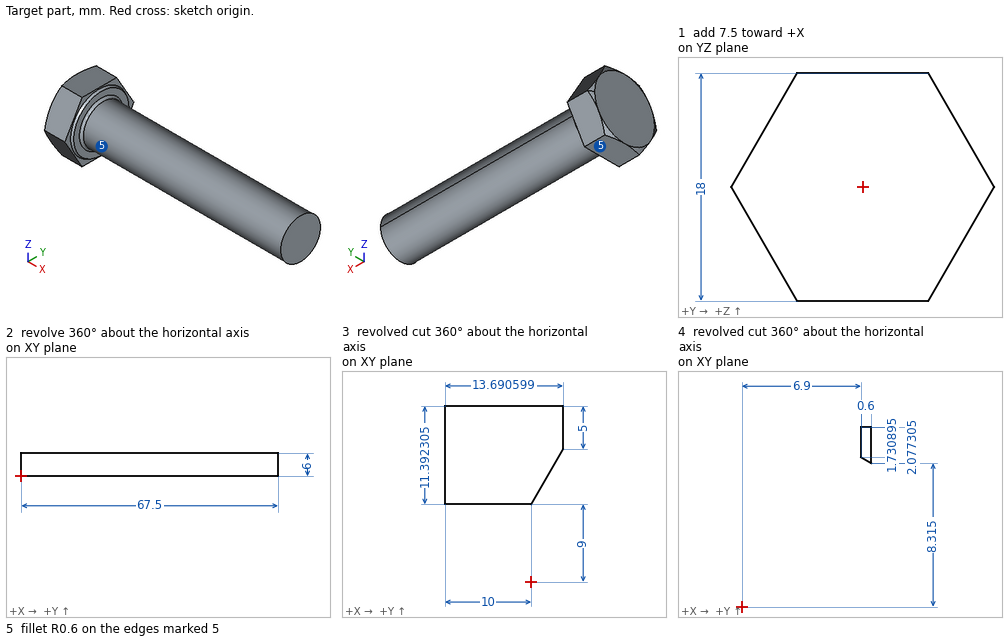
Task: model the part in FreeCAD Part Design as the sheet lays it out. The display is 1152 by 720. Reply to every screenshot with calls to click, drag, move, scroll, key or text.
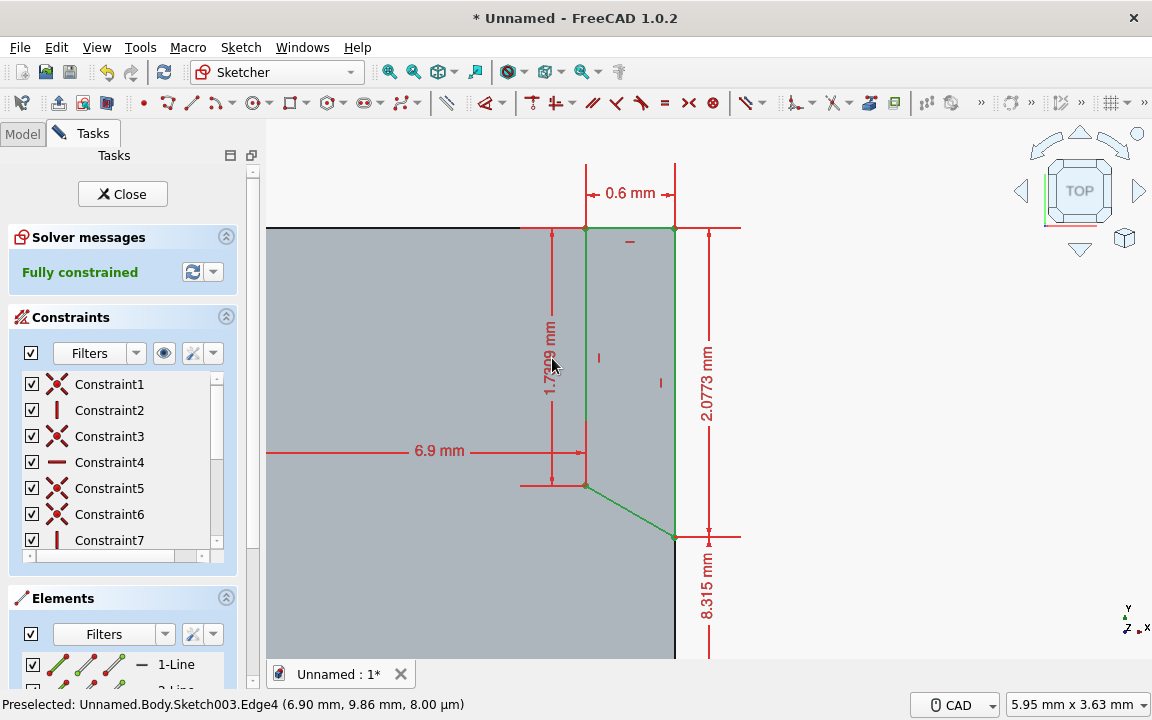
click(123, 194)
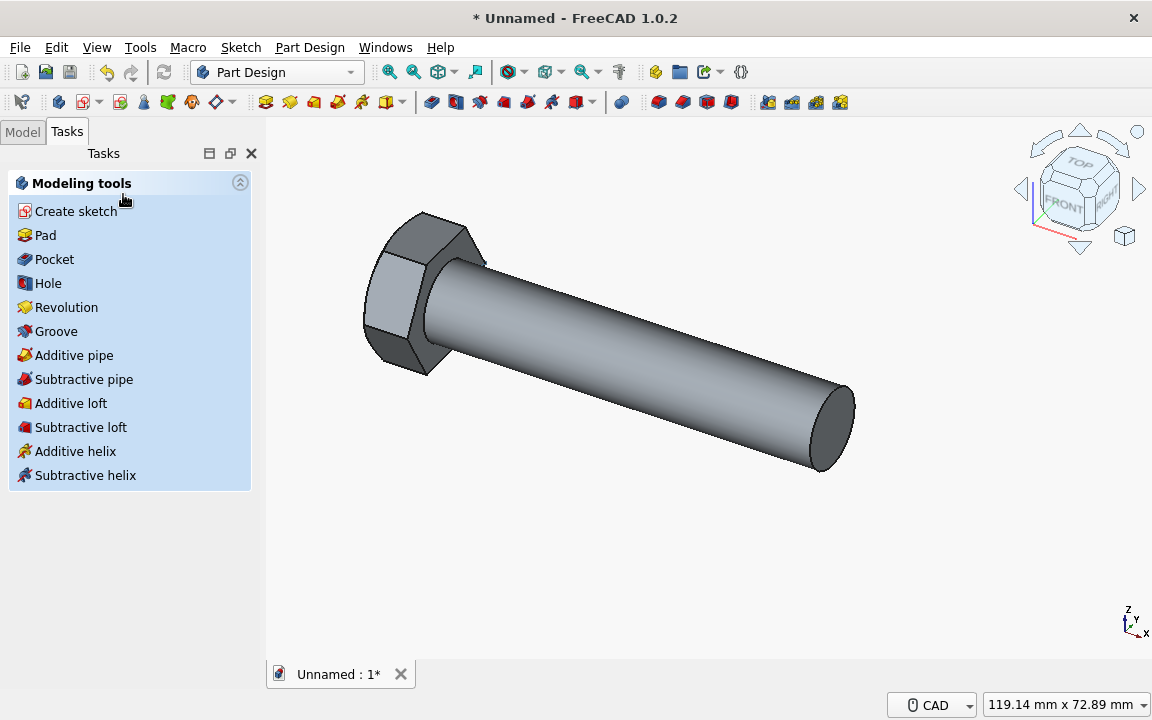
click(480, 102)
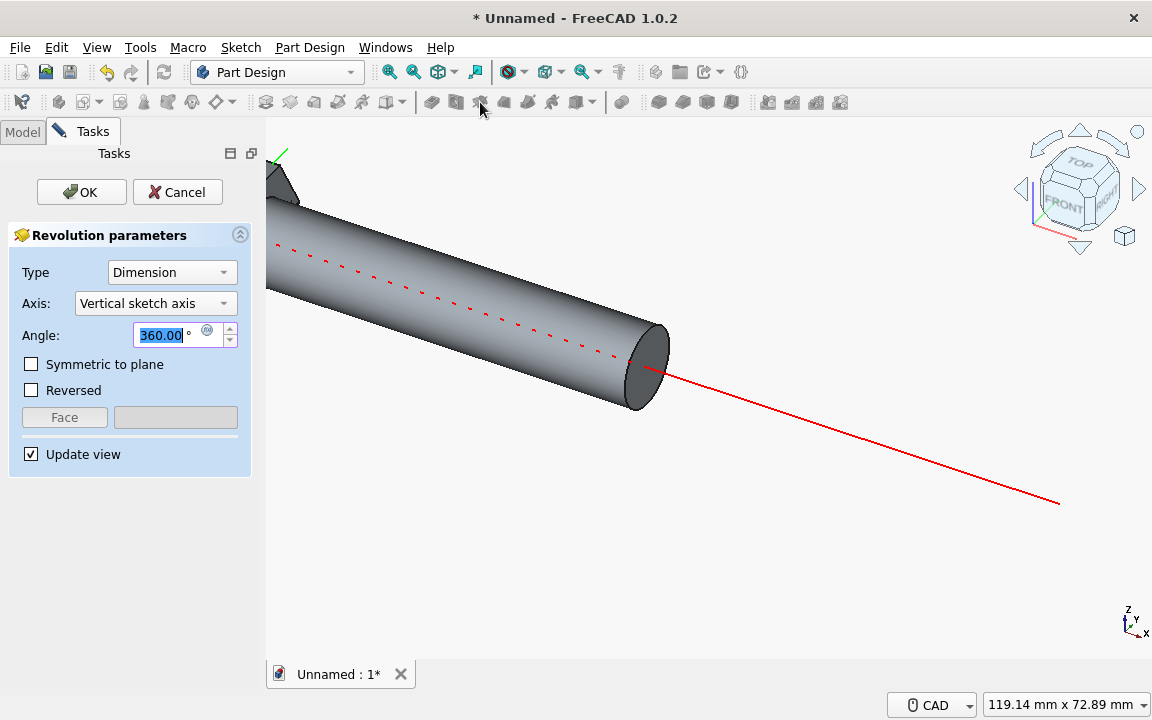
click(156, 304)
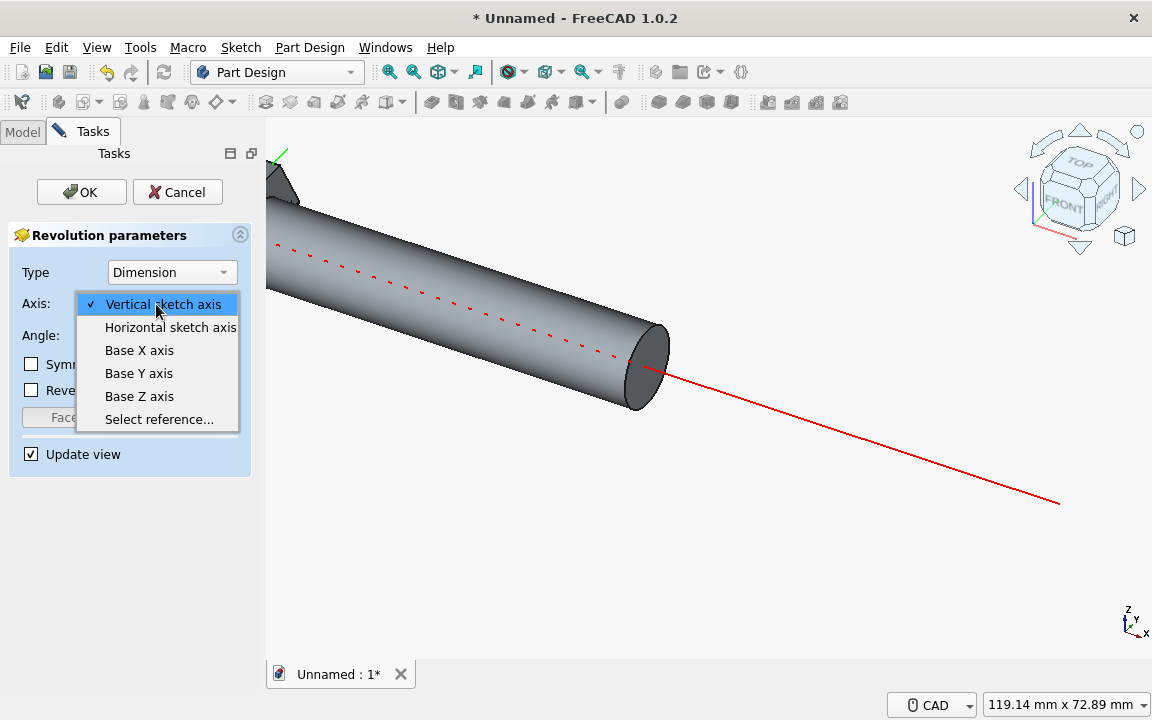
click(156, 328)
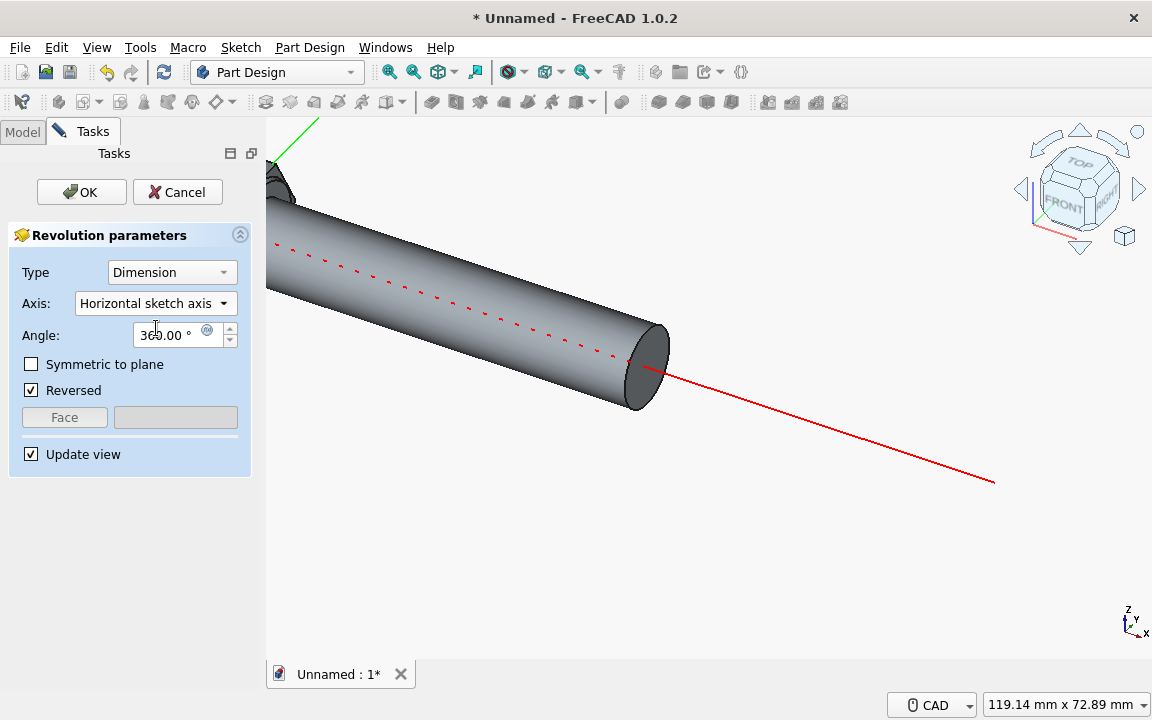
click(82, 192)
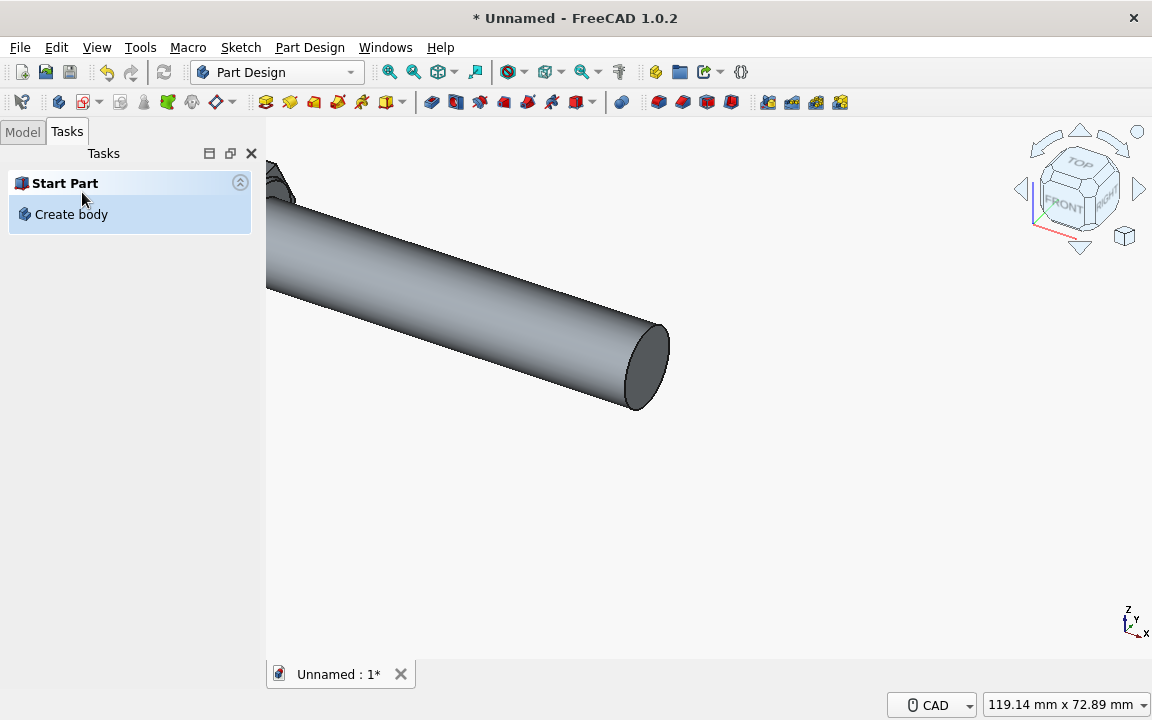
click(390, 72)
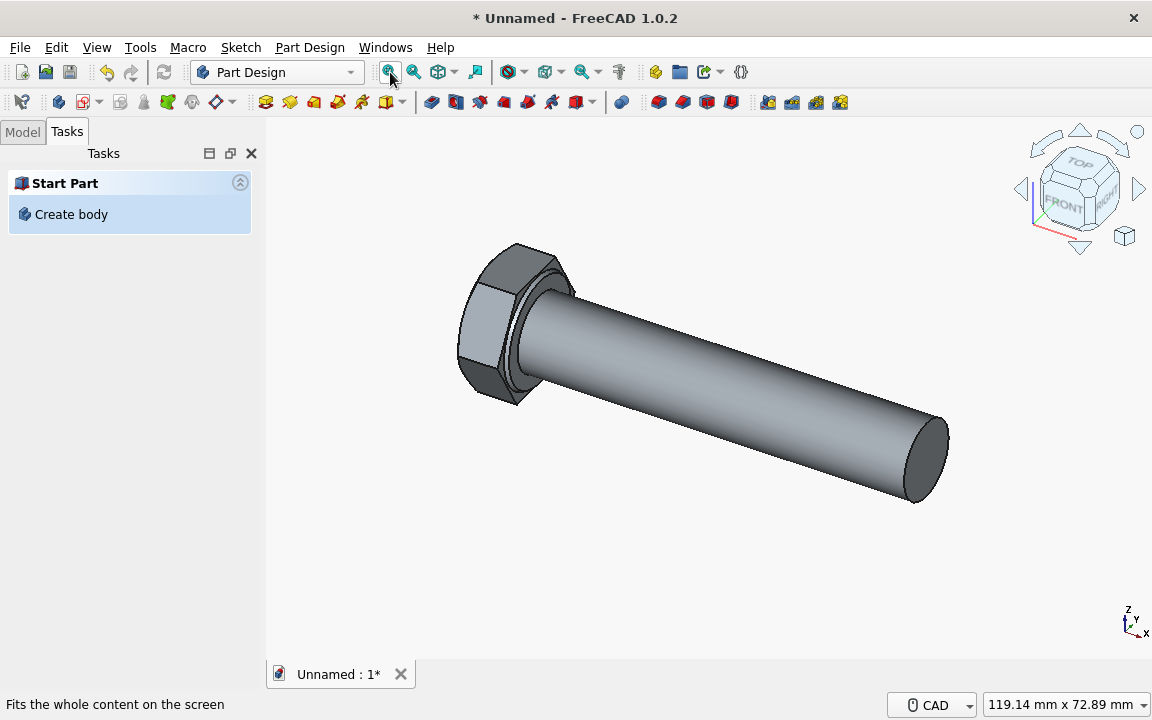
key(0)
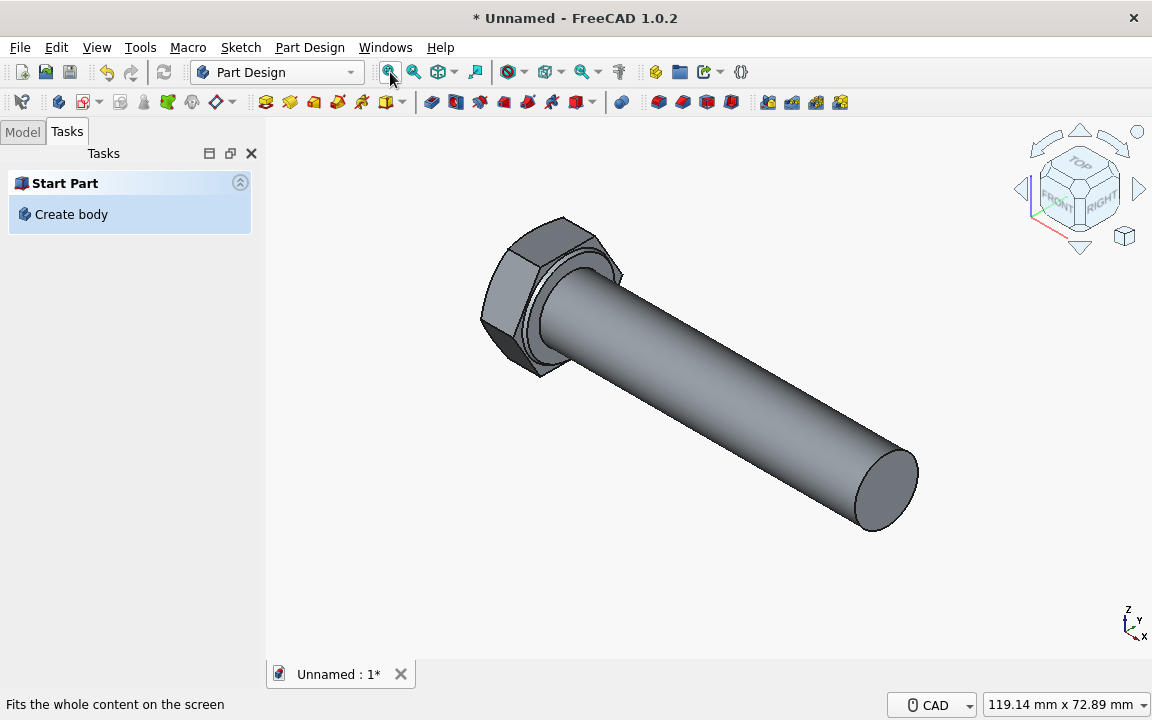
key(2)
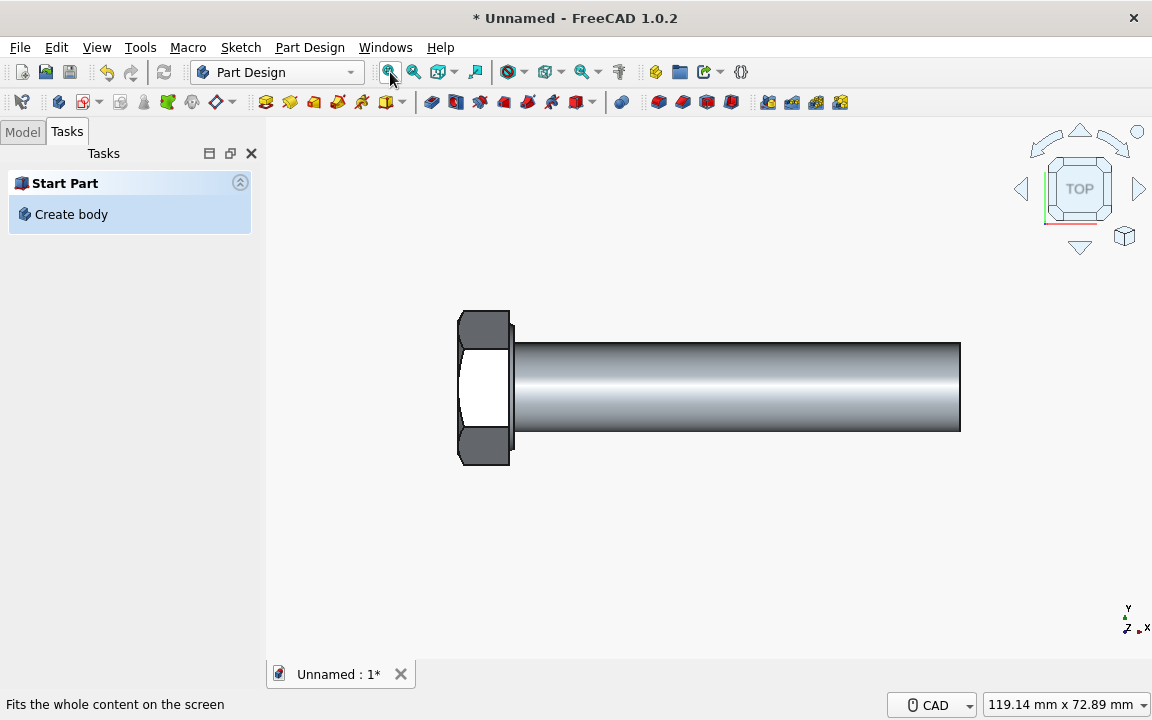
key(1)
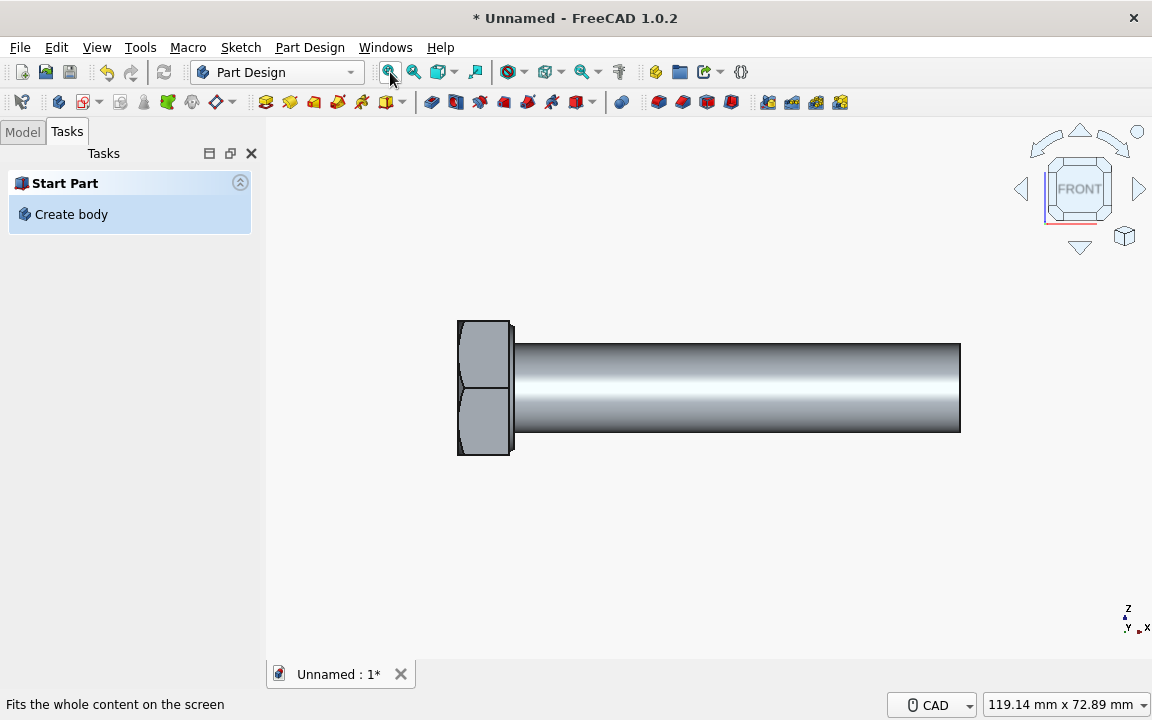
key(3)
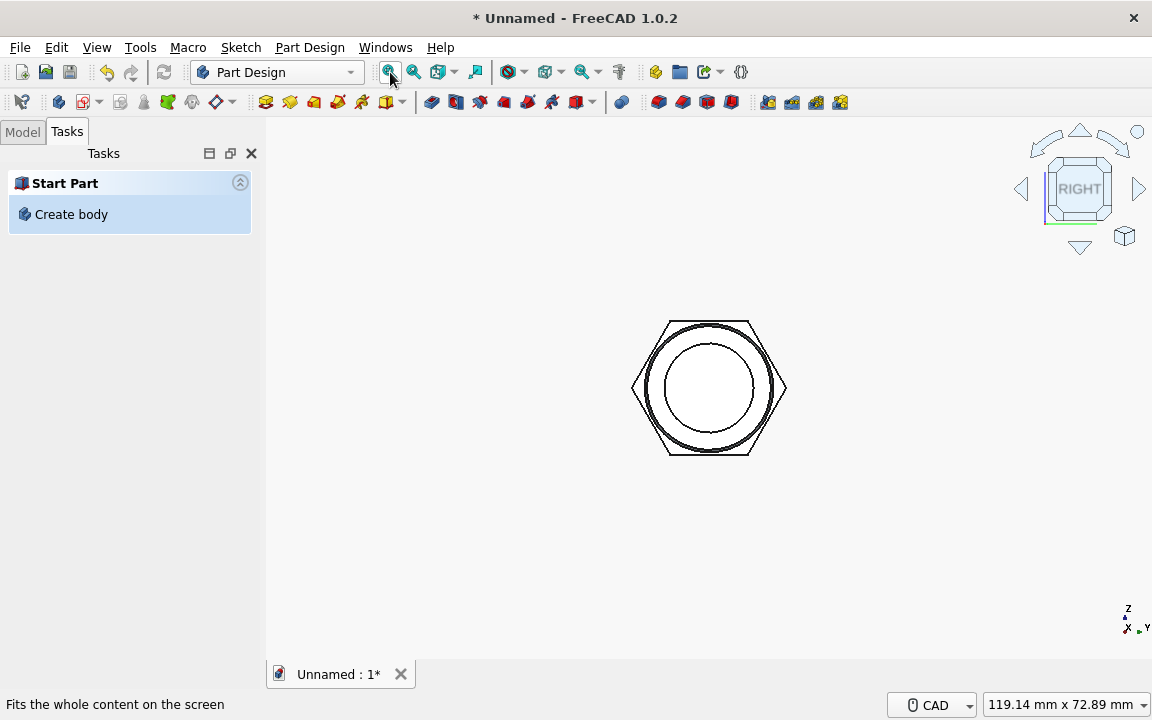
click(390, 72)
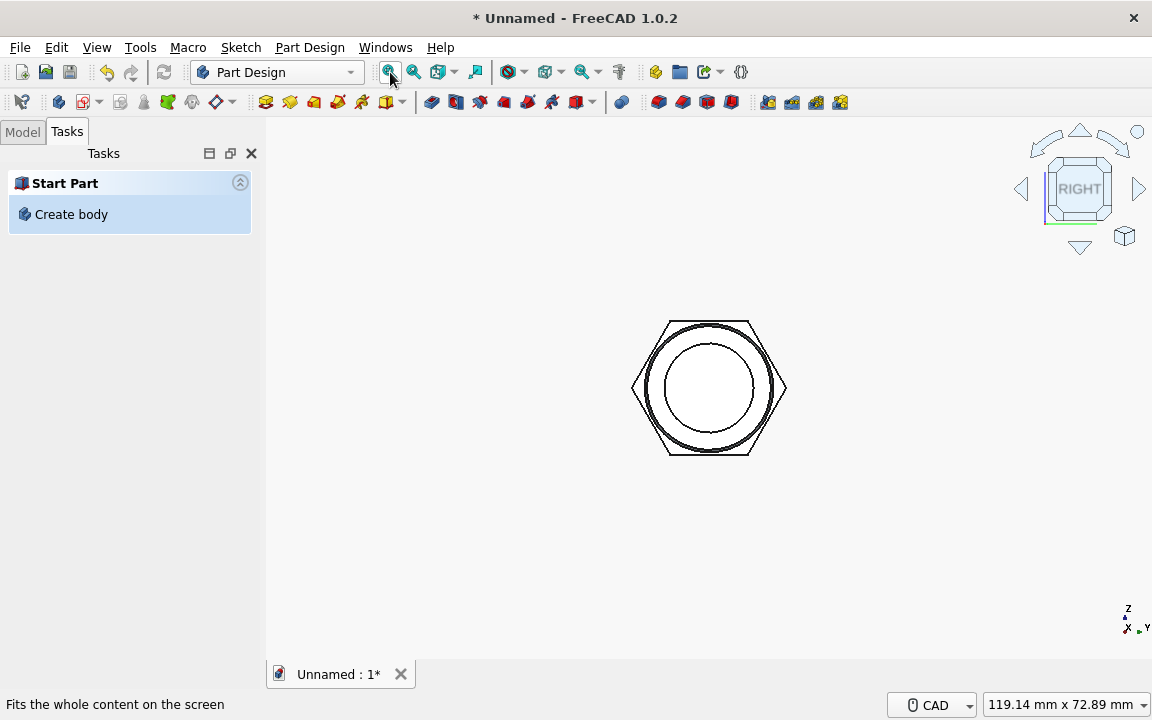
key(5)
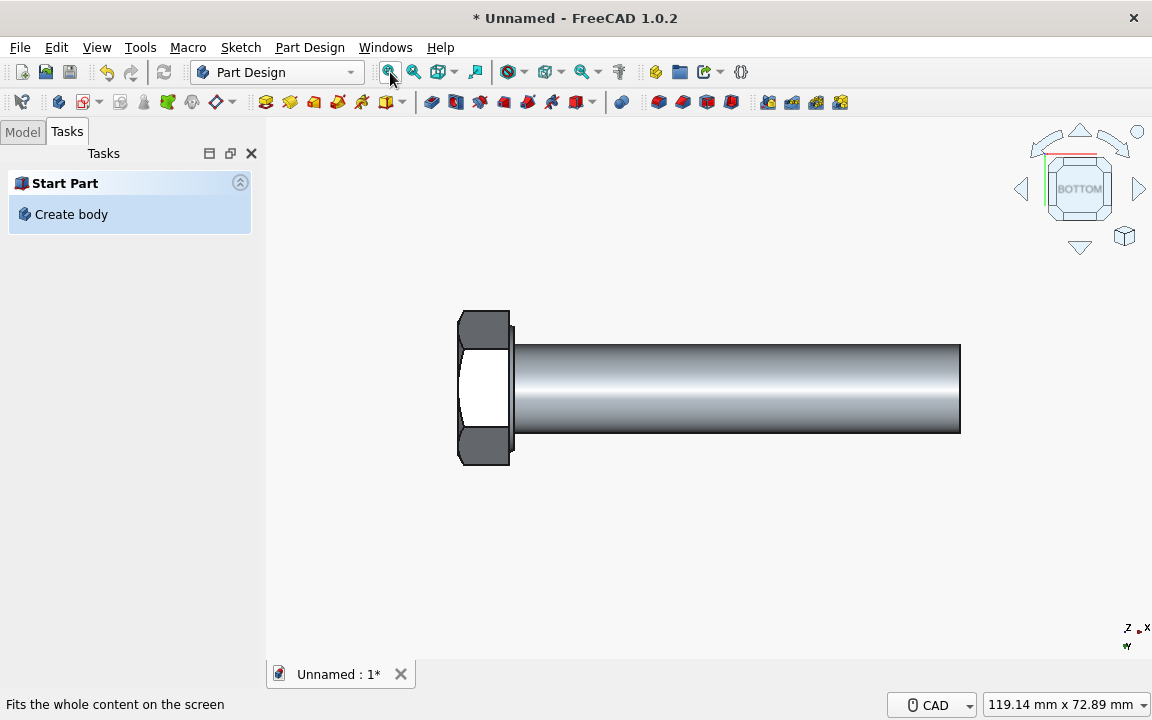
key(4)